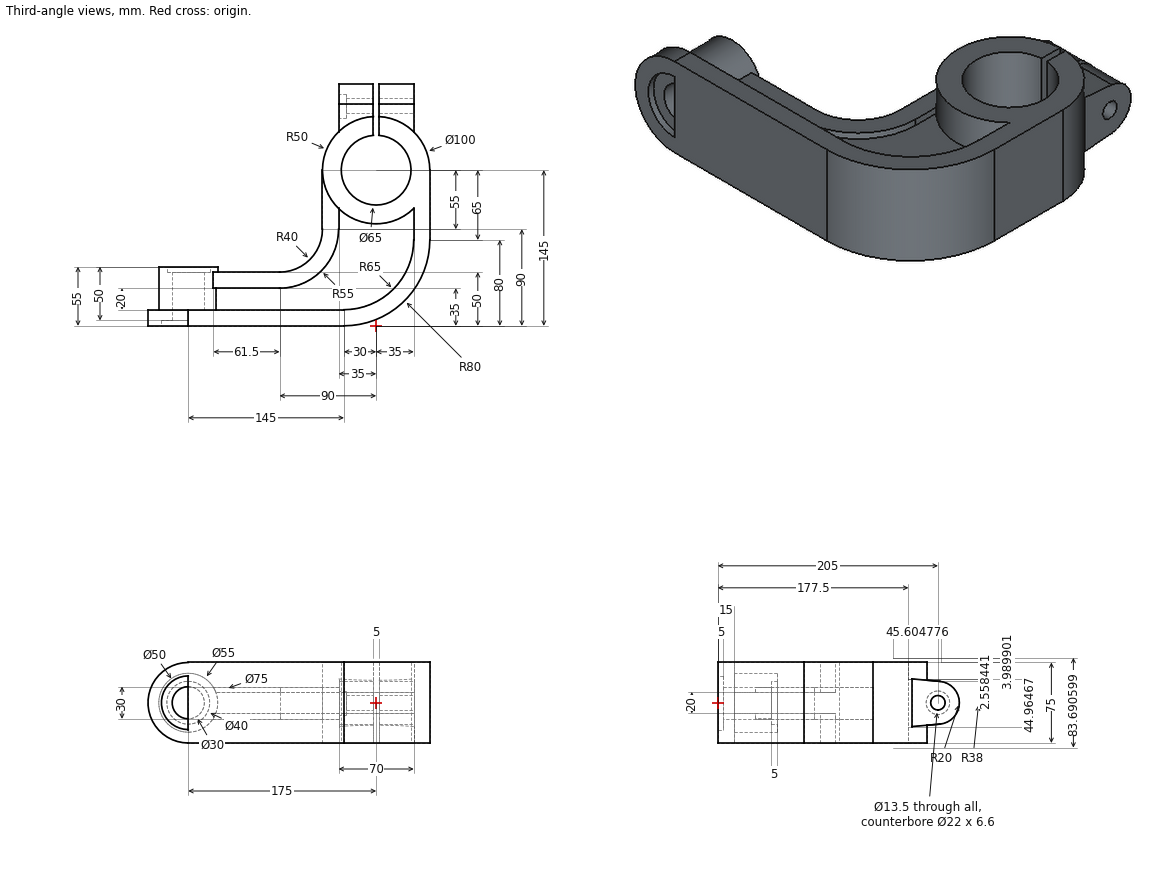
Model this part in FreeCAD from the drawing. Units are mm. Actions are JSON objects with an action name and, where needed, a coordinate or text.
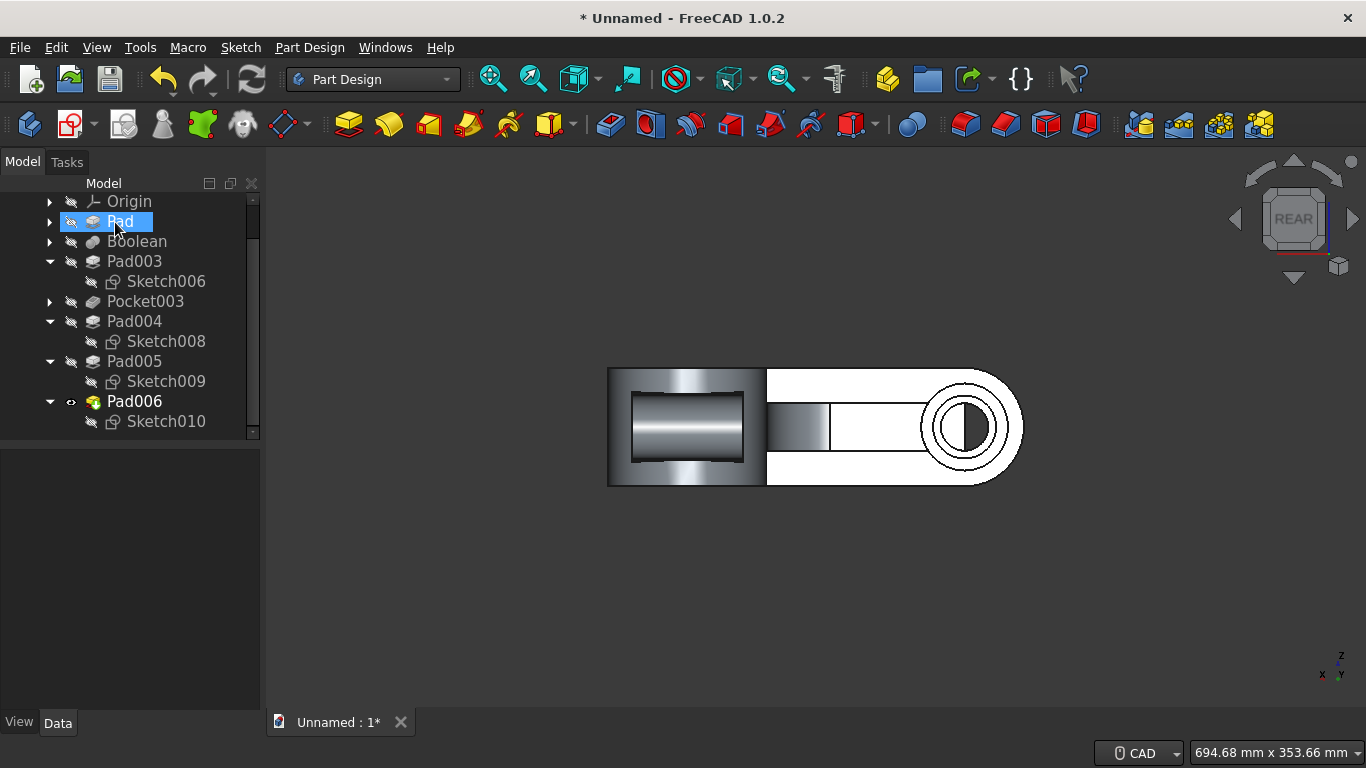
{"action": "left_click", "coordinate": [70, 124]}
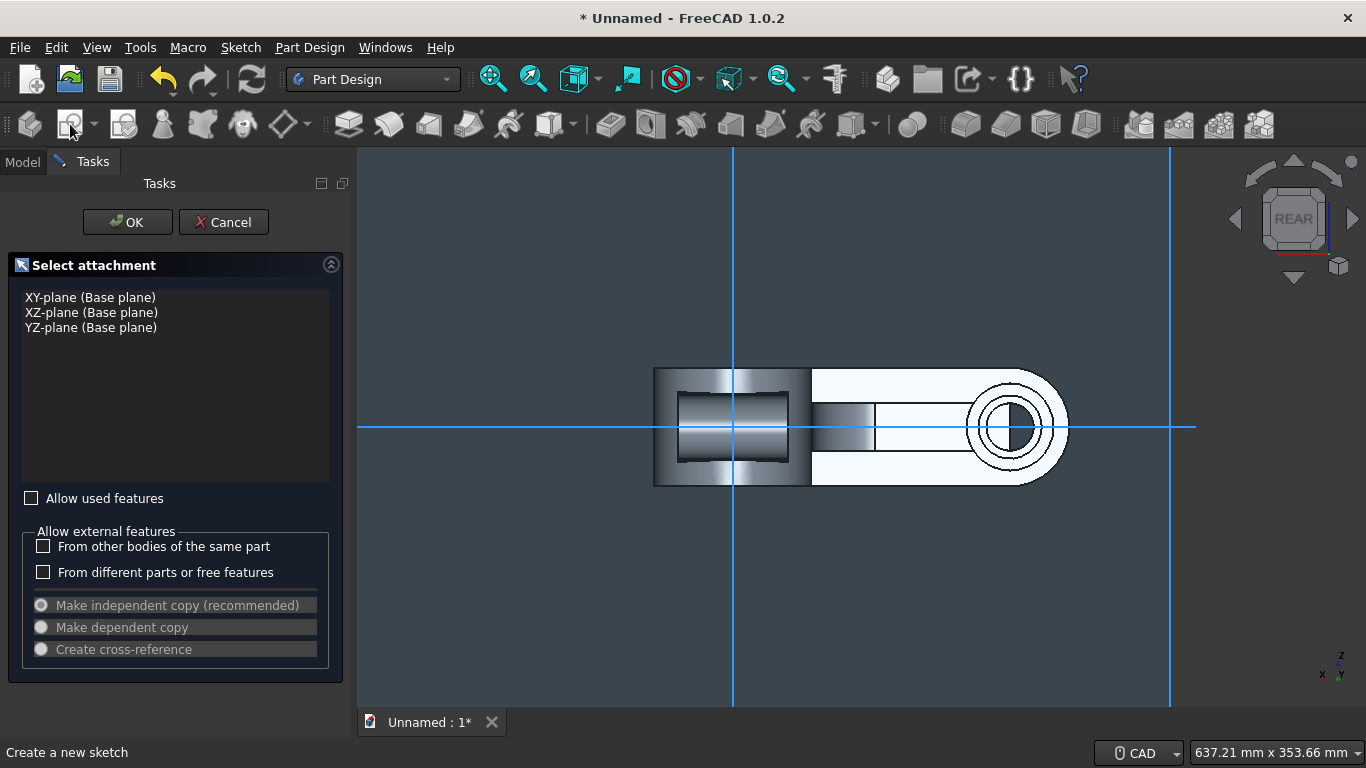
{"action": "left_click", "coordinate": [82, 328]}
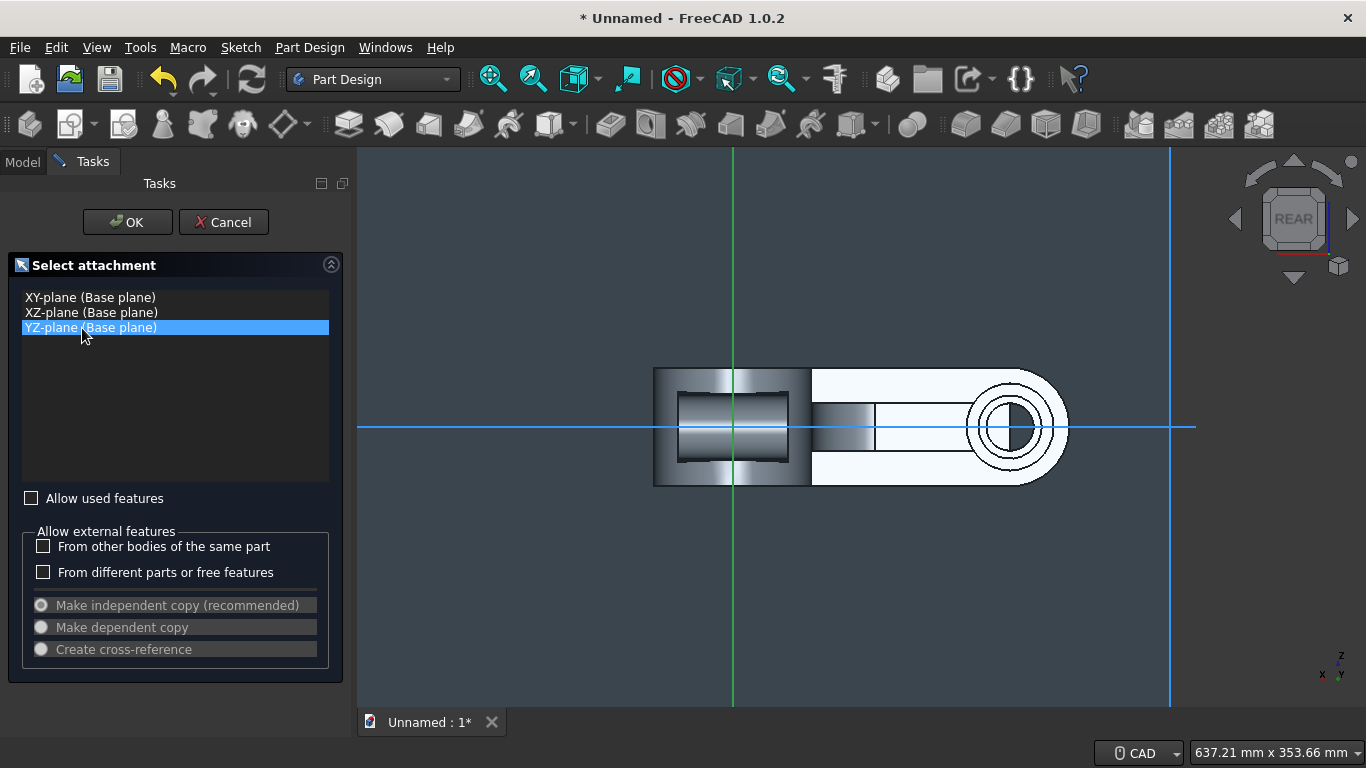
{"action": "left_click", "coordinate": [128, 222]}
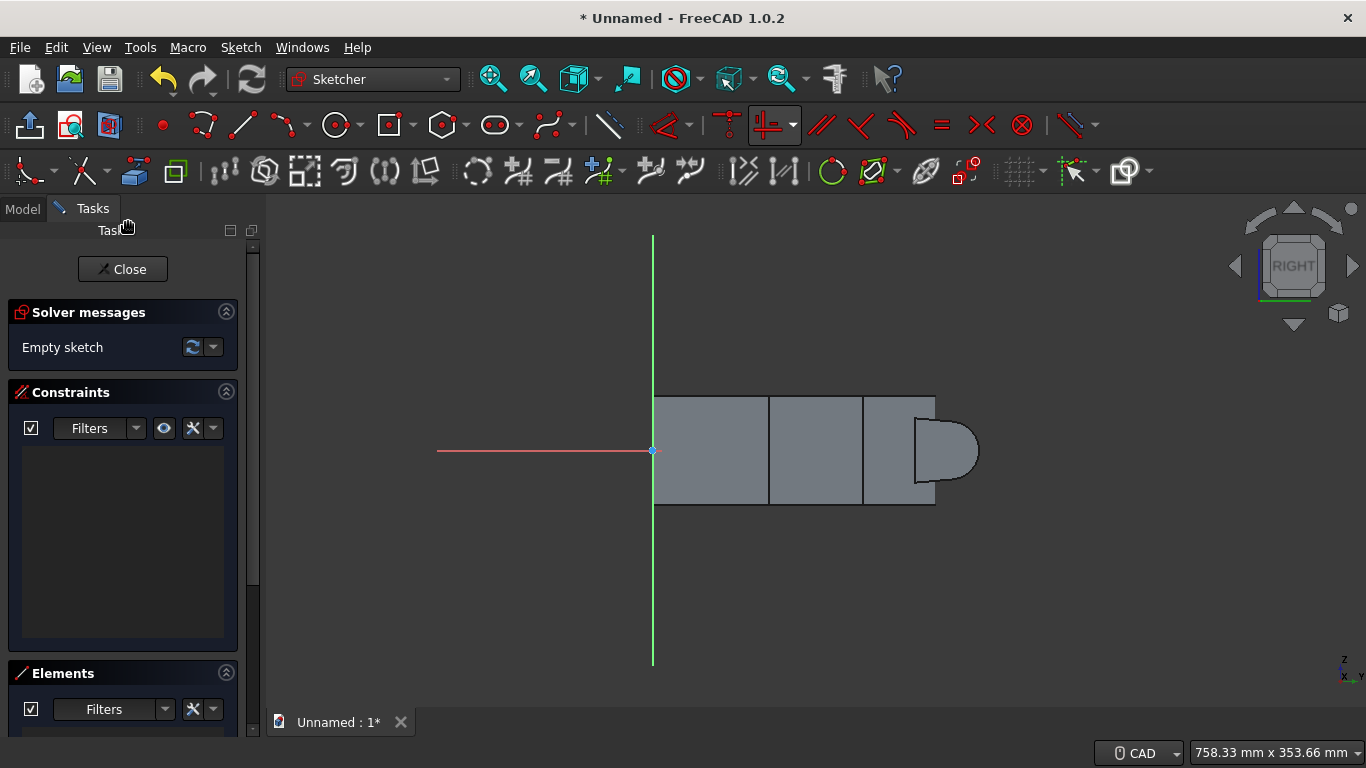
{"action": "key", "text": "q s"}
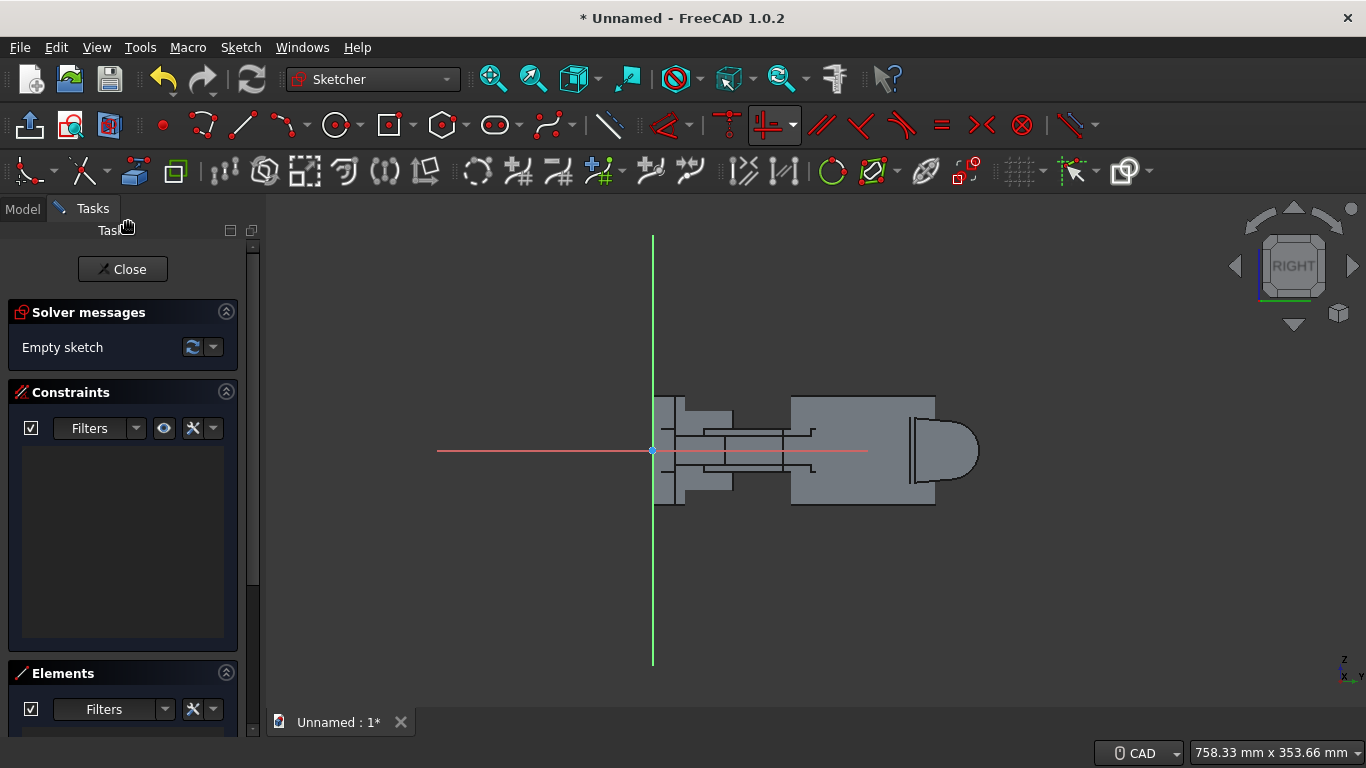
{"action": "scroll", "coordinate": [1063, 450], "scroll_direction": "up", "scroll_amount": 5}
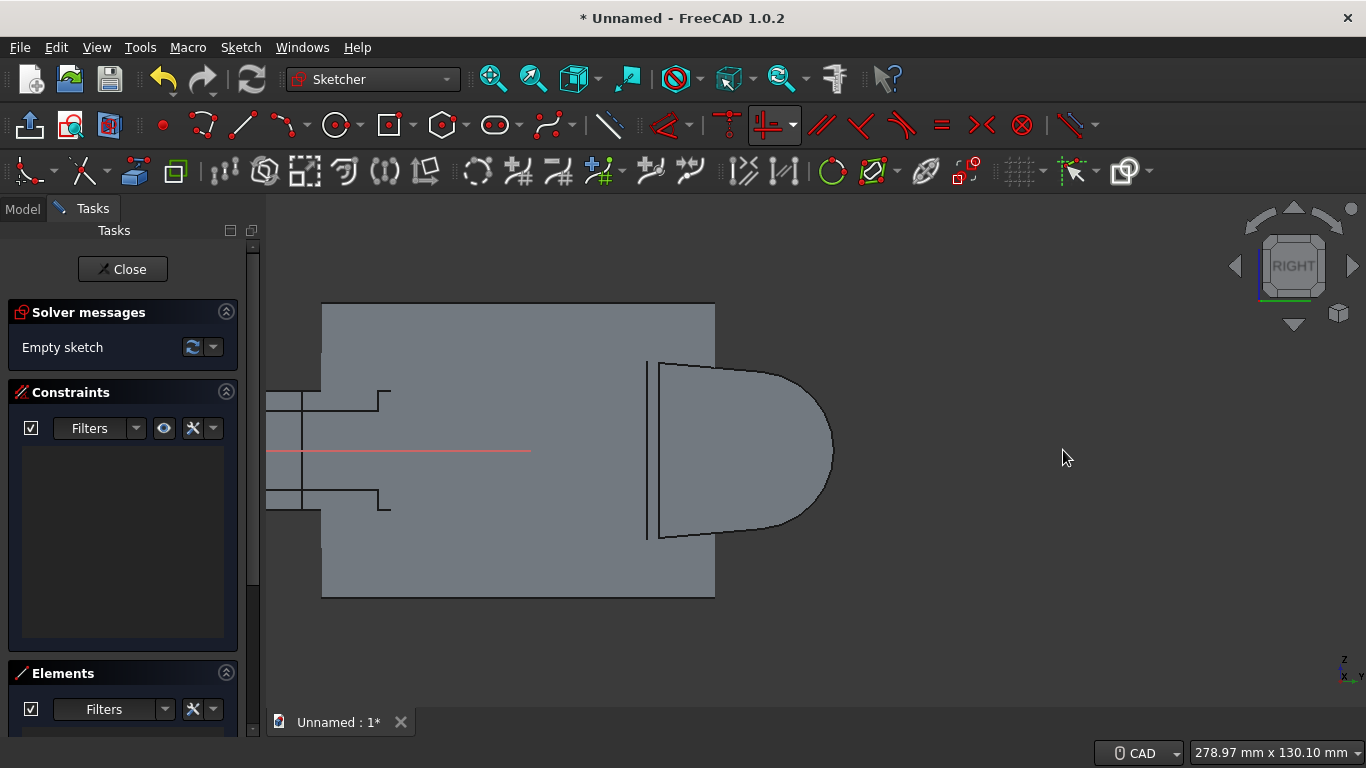
{"action": "left_click", "coordinate": [204, 126]}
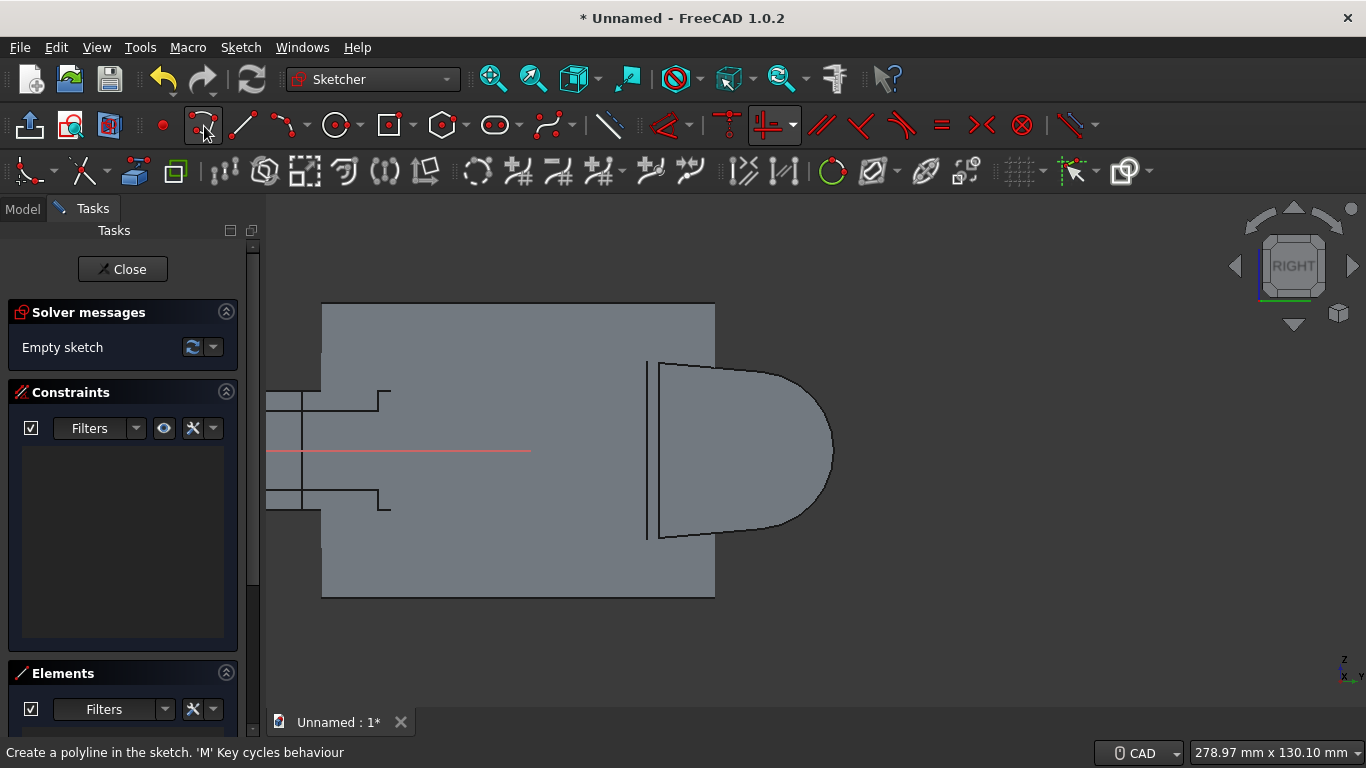
{"action": "left_click", "coordinate": [768, 301]}
{"action": "left_click", "coordinate": [588, 286]}
{"action": "left_click", "coordinate": [588, 615]}
{"action": "left_click", "coordinate": [768, 600]}
{"action": "right_click", "coordinate": [768, 600]}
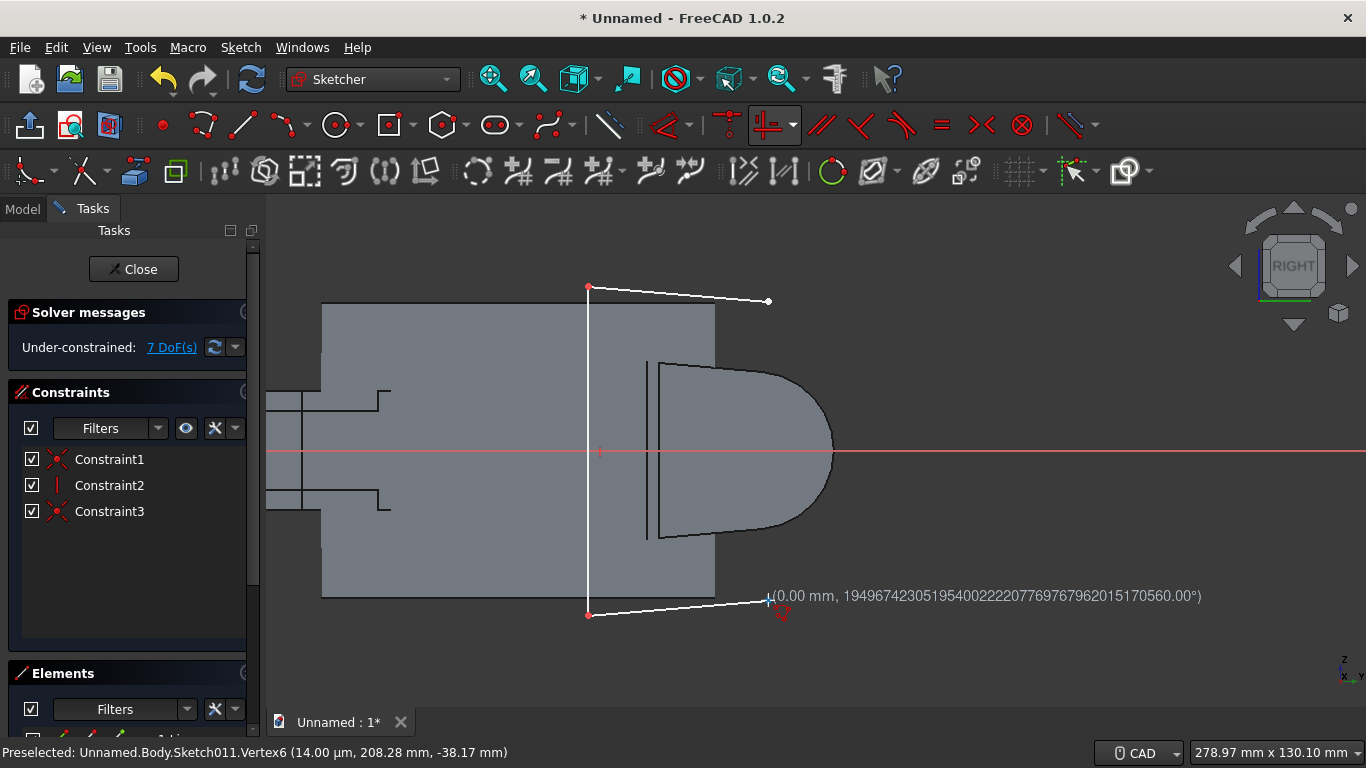
{"action": "key", "text": "g 3 a"}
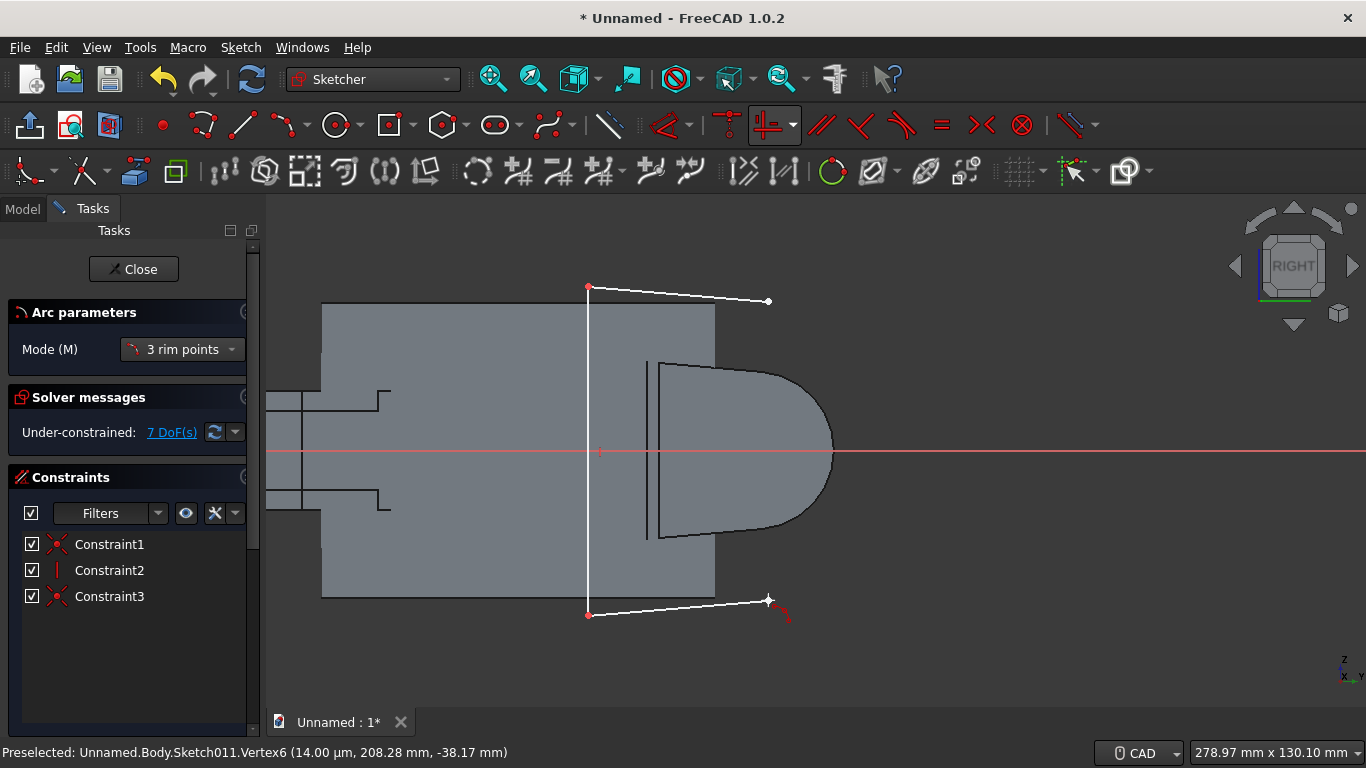
{"action": "left_click", "coordinate": [768, 601]}
{"action": "left_click", "coordinate": [768, 302]}
{"action": "left_click", "coordinate": [898, 494]}
{"action": "key", "text": "Escape"}